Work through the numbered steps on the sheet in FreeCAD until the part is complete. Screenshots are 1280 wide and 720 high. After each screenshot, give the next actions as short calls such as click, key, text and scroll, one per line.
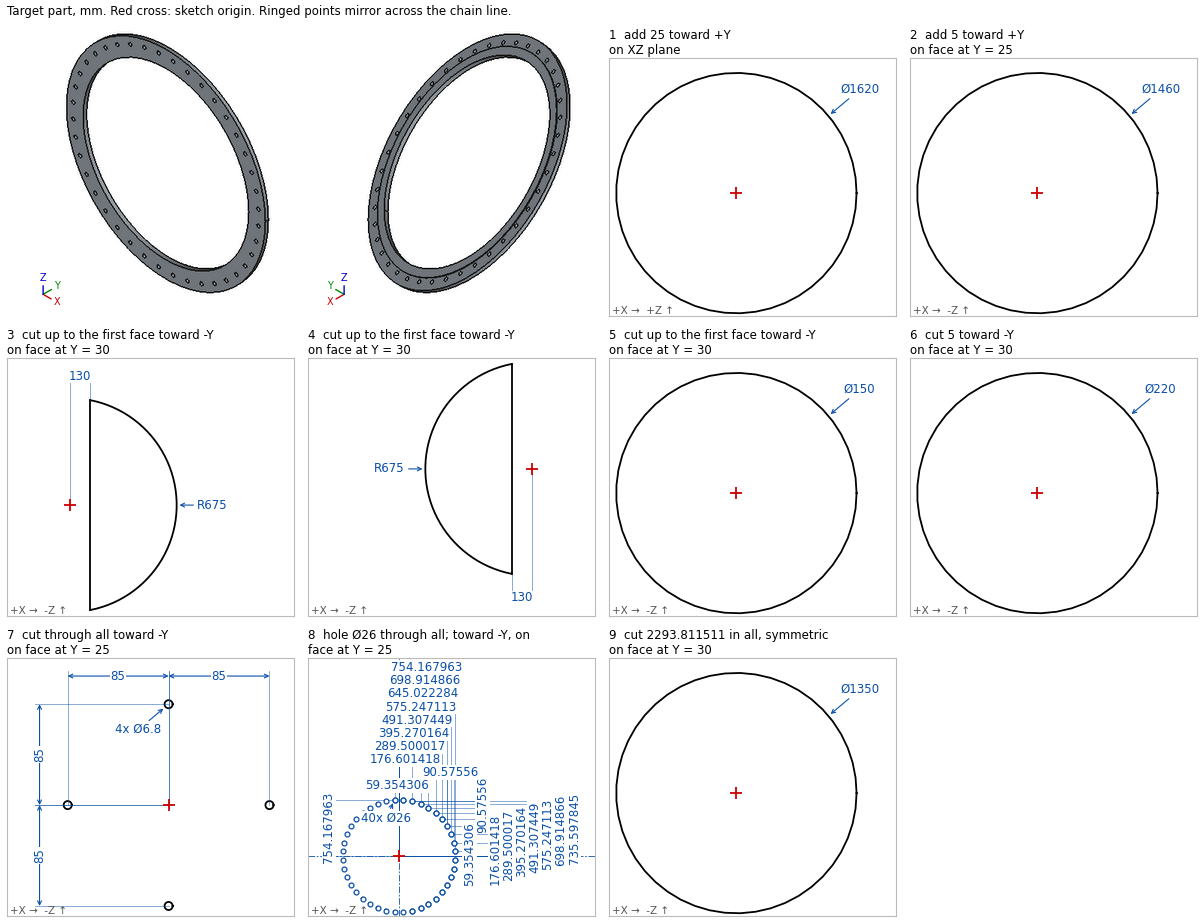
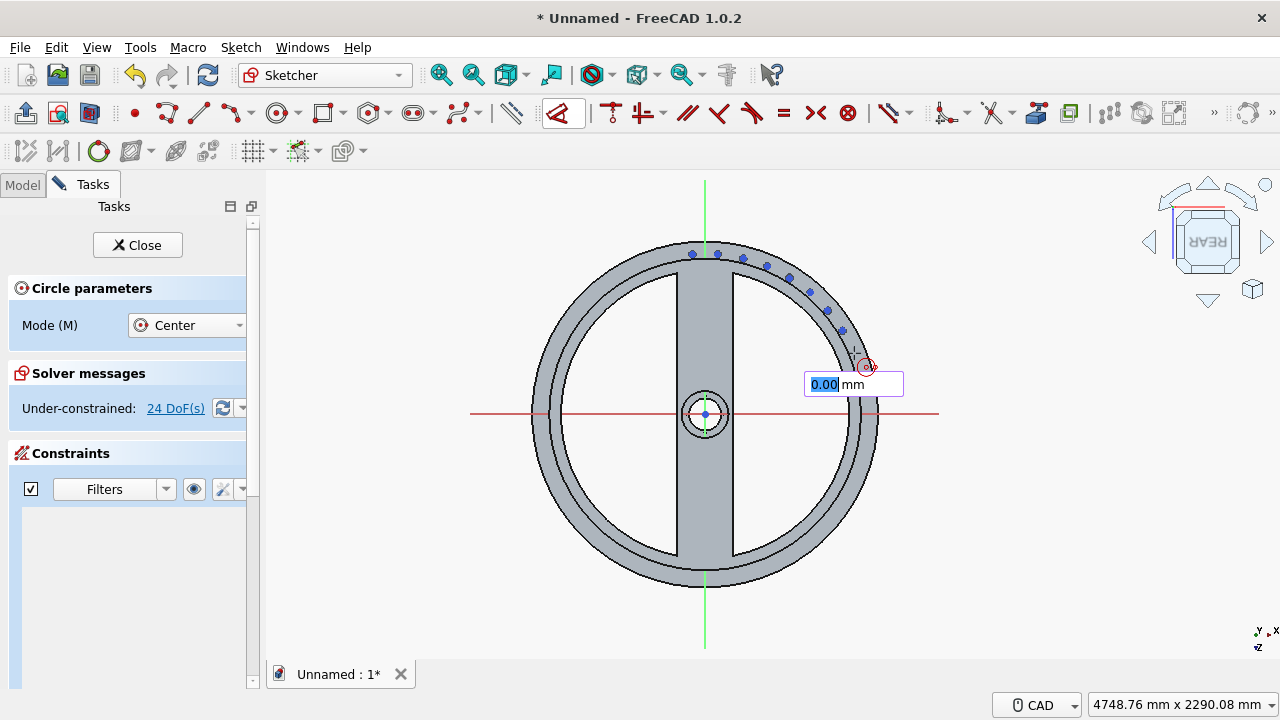
scroll(856, 351, up, 9)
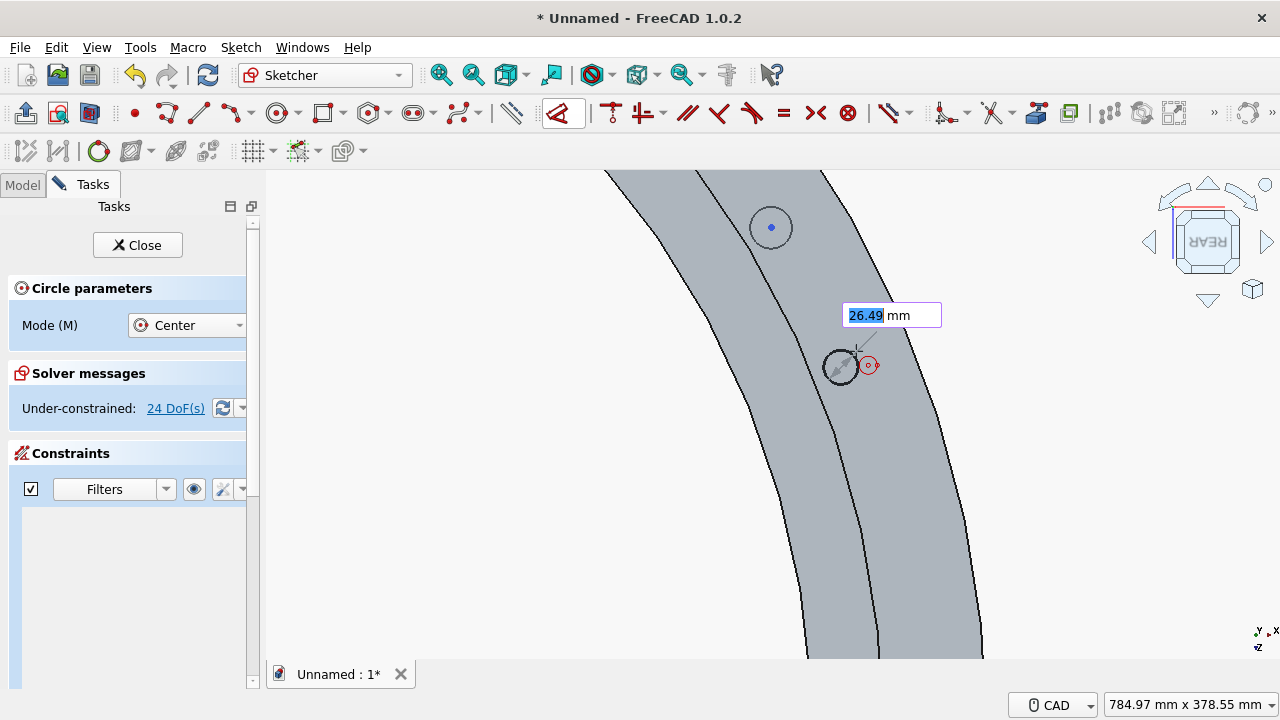
click(855, 347)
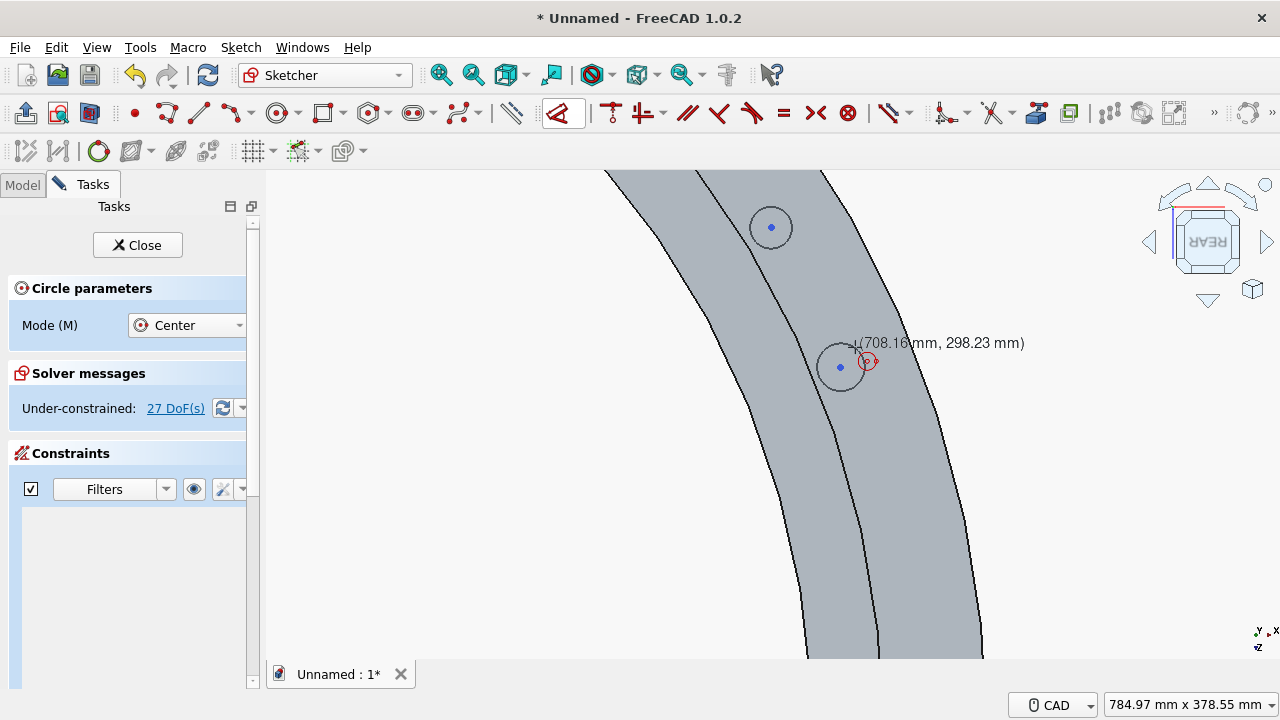
scroll(890, 505, up, 2)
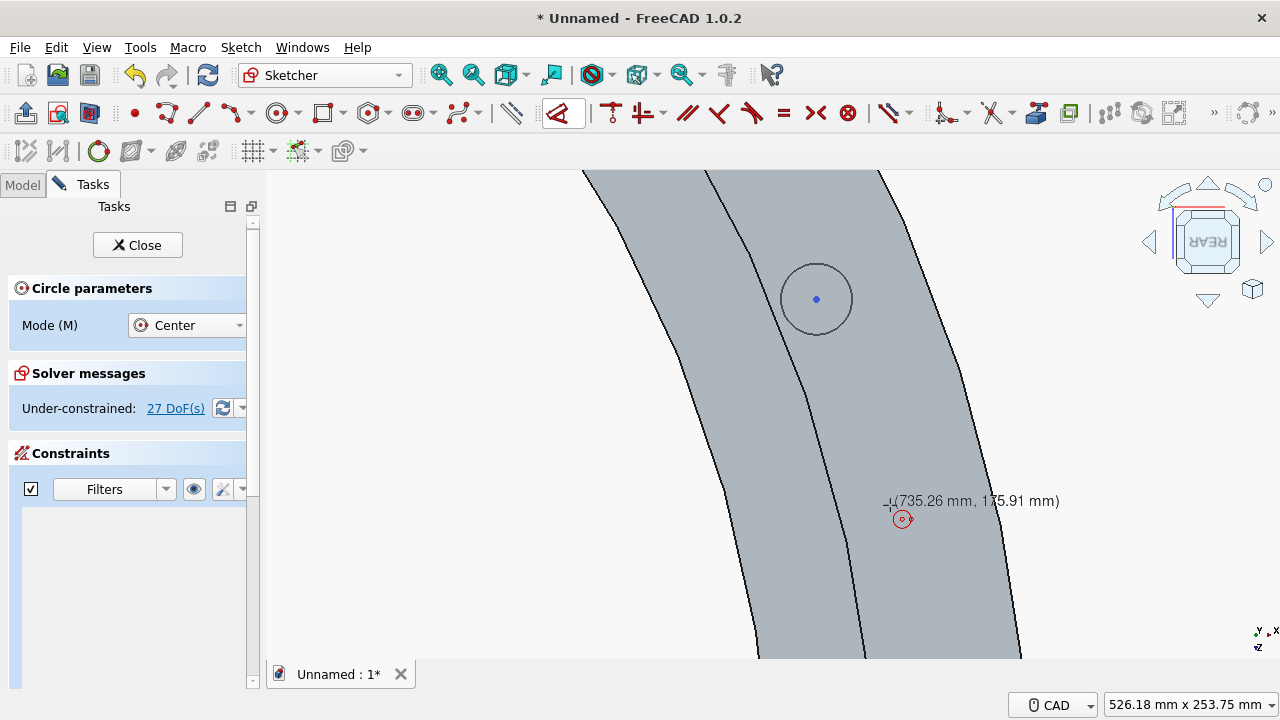
scroll(858, 361, down, 11)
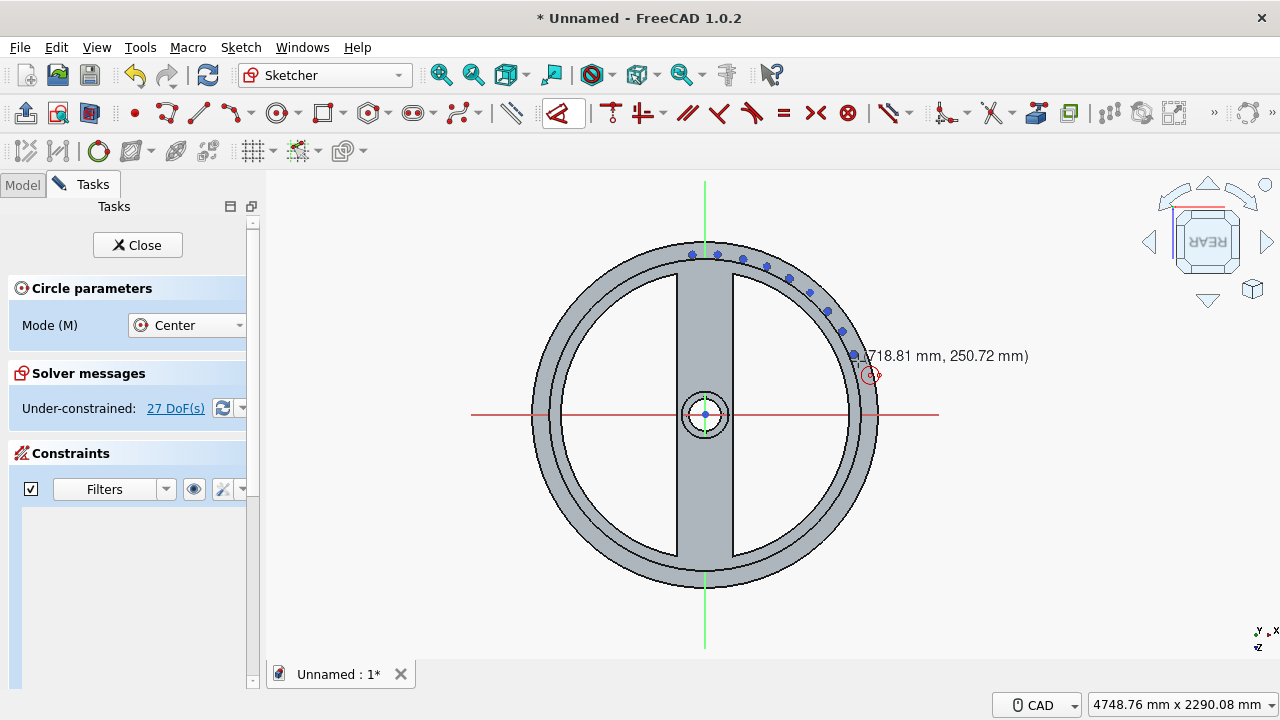
click(862, 377)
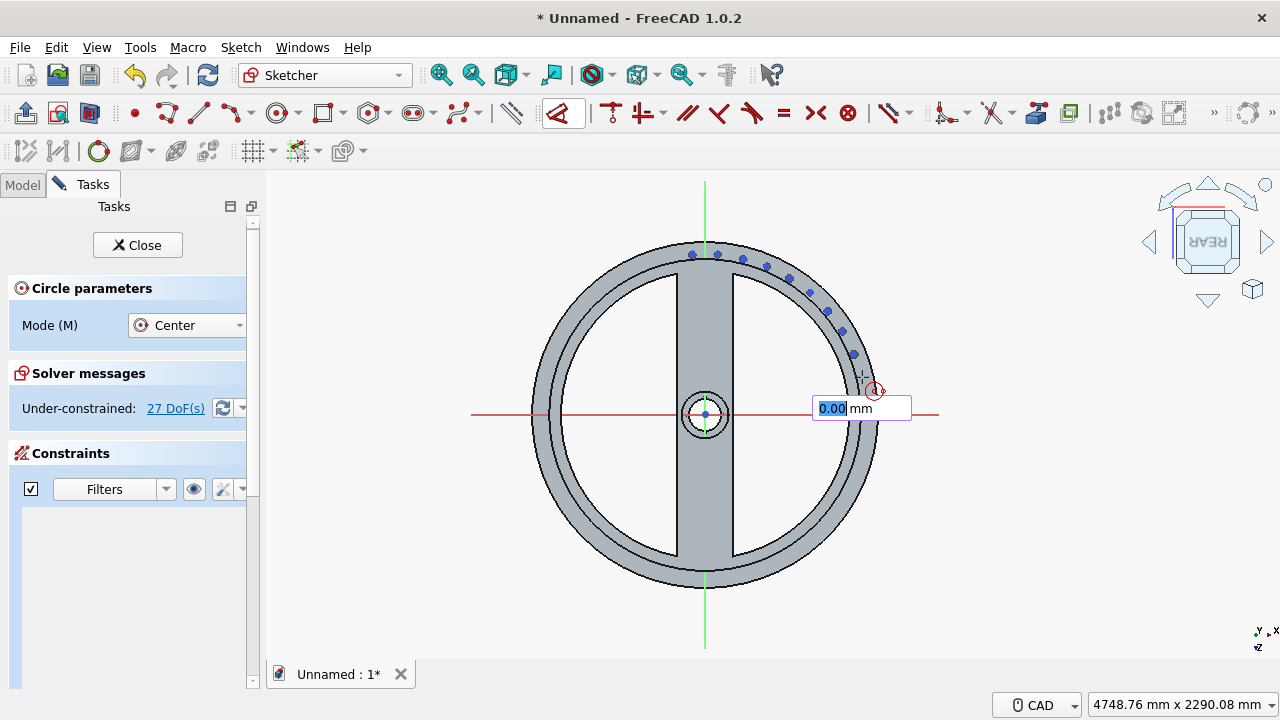
scroll(864, 375, up, 9)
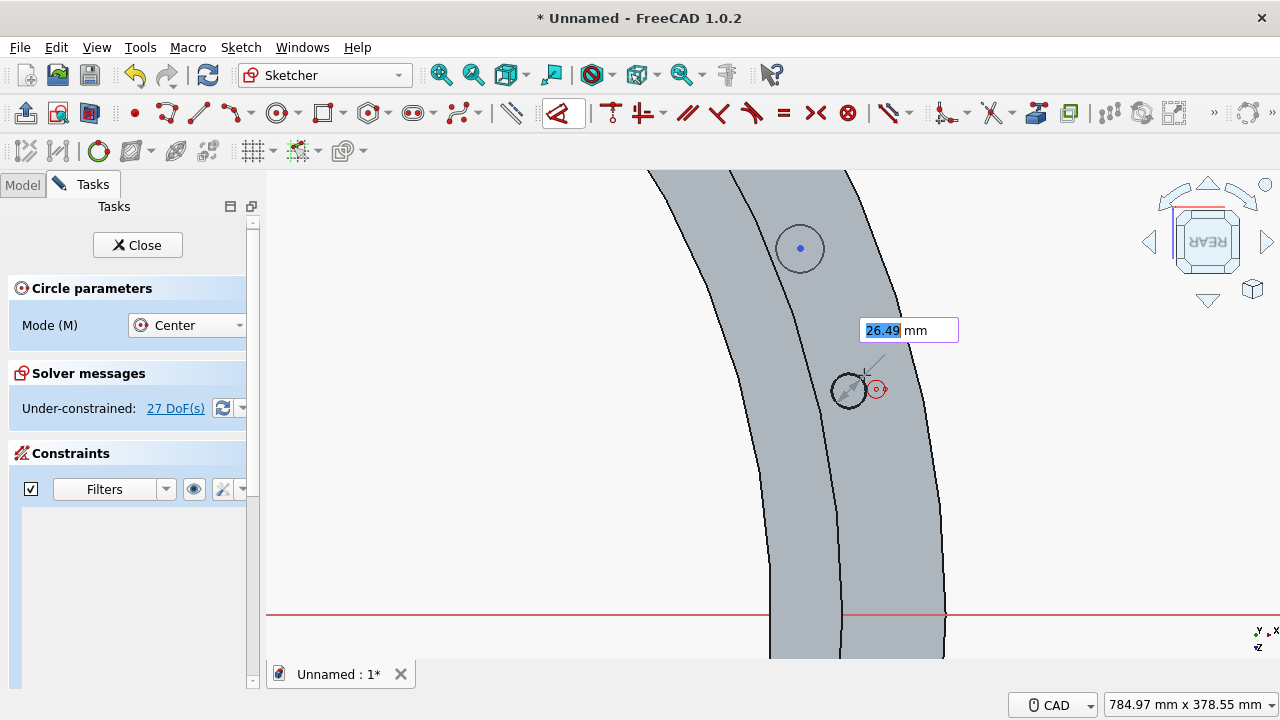
click(861, 375)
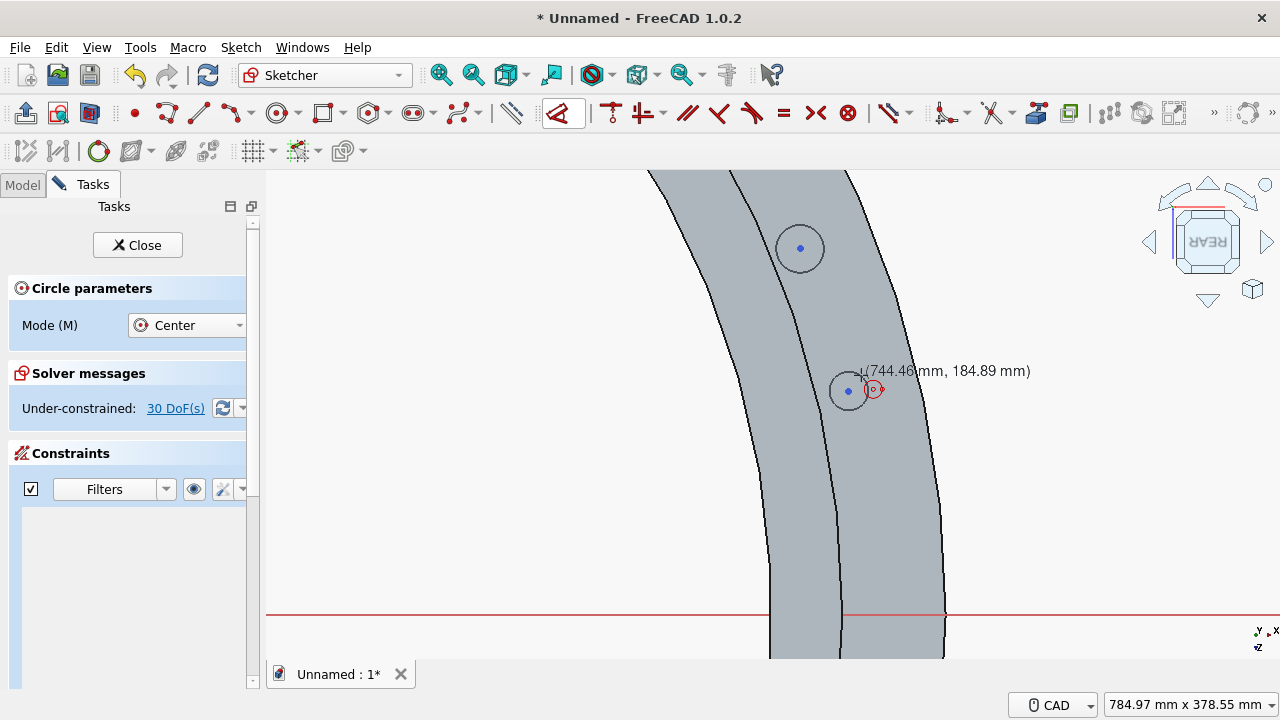
scroll(874, 538, up, 2)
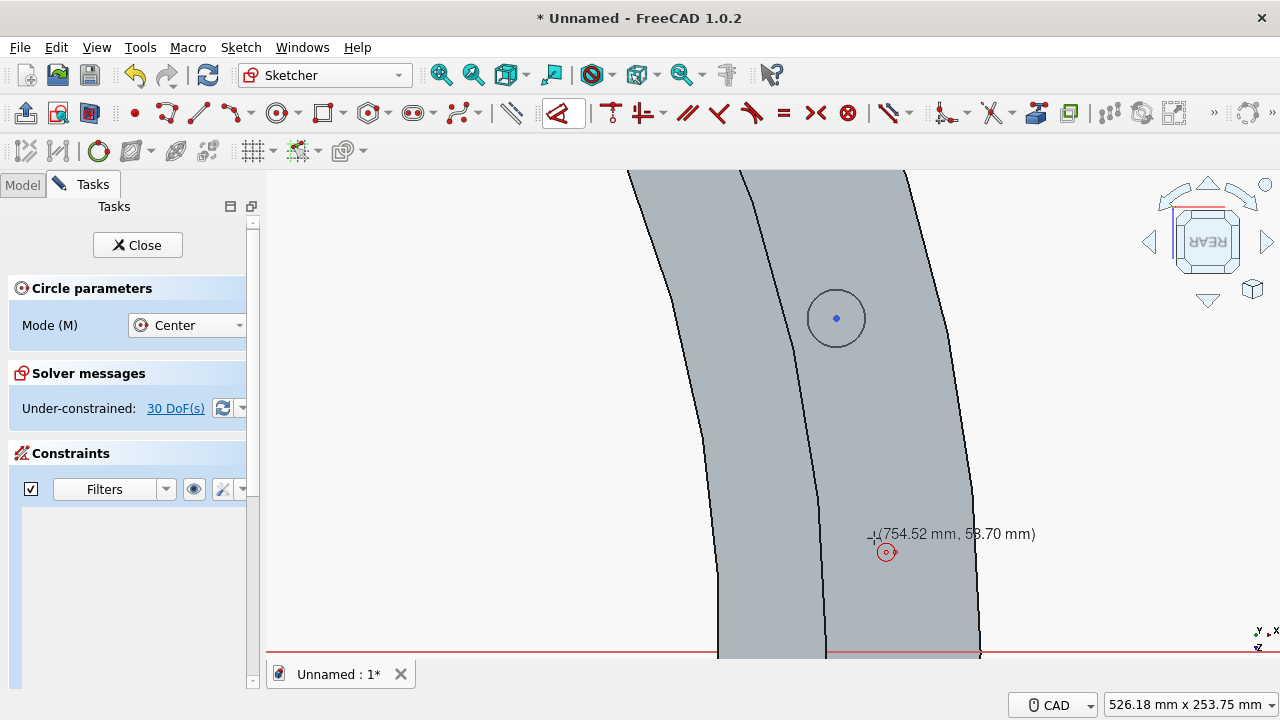
scroll(865, 385, down, 11)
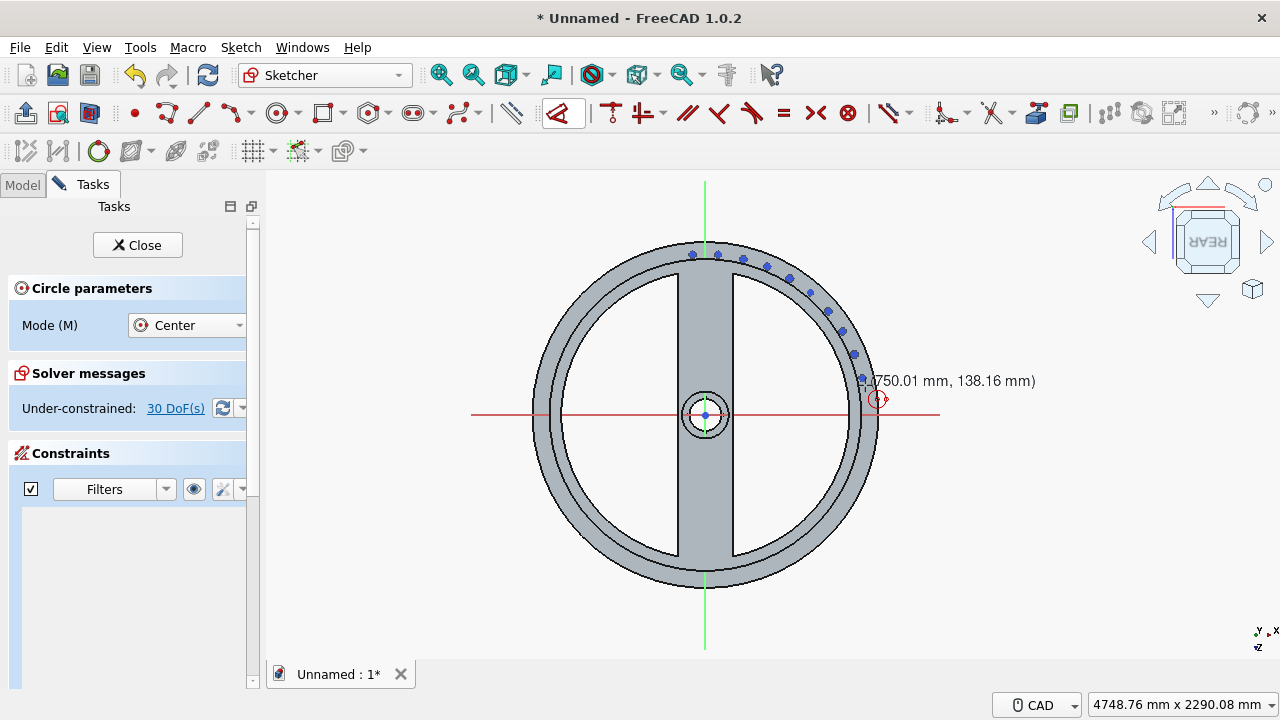
scroll(866, 402, up, 2)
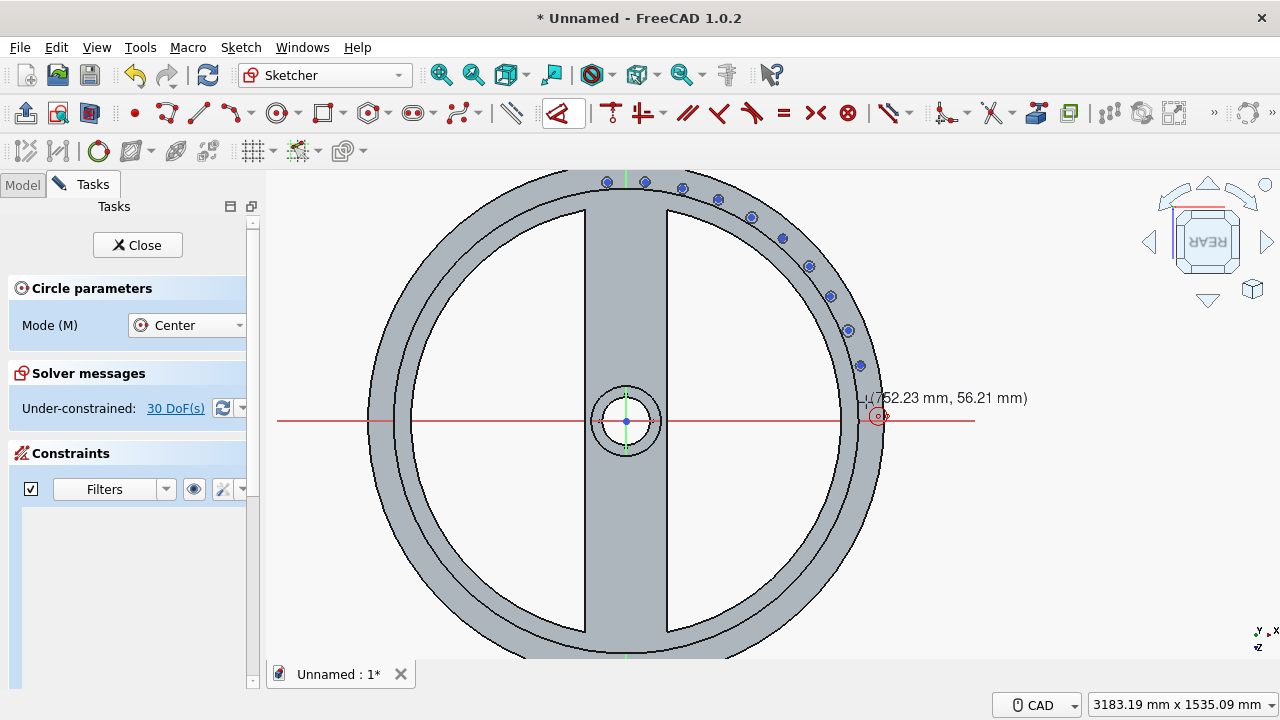
click(866, 402)